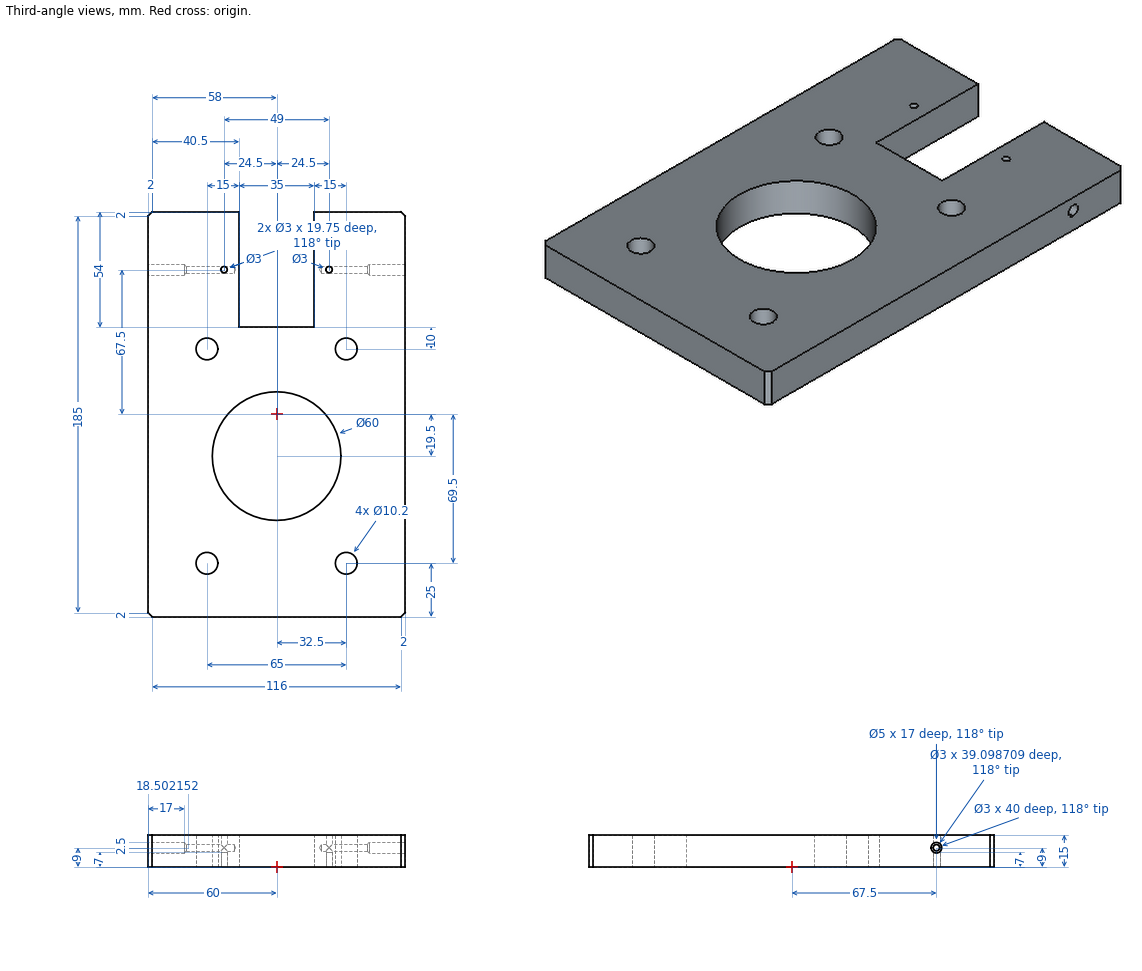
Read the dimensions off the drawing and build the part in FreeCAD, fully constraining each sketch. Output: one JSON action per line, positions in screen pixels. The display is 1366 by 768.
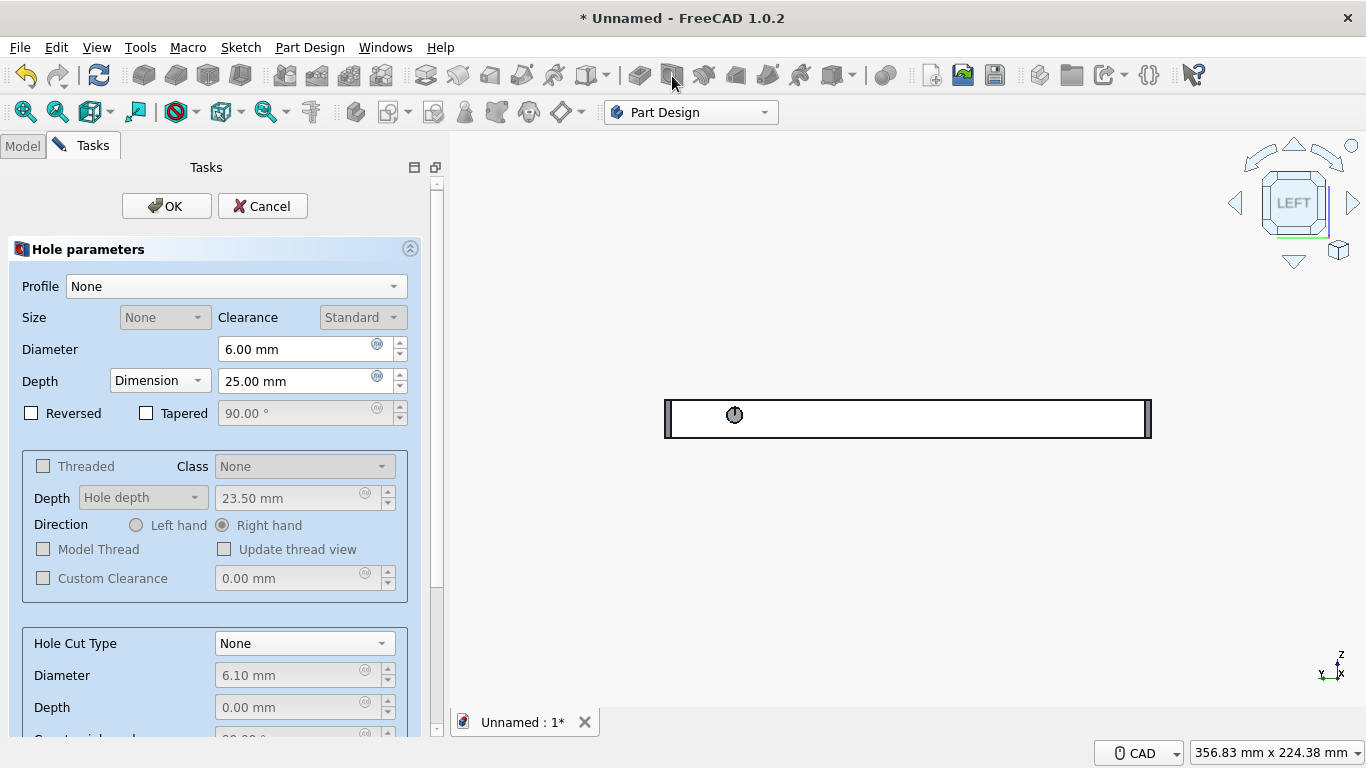
{"action": "triple_click", "coordinate": [305, 349]}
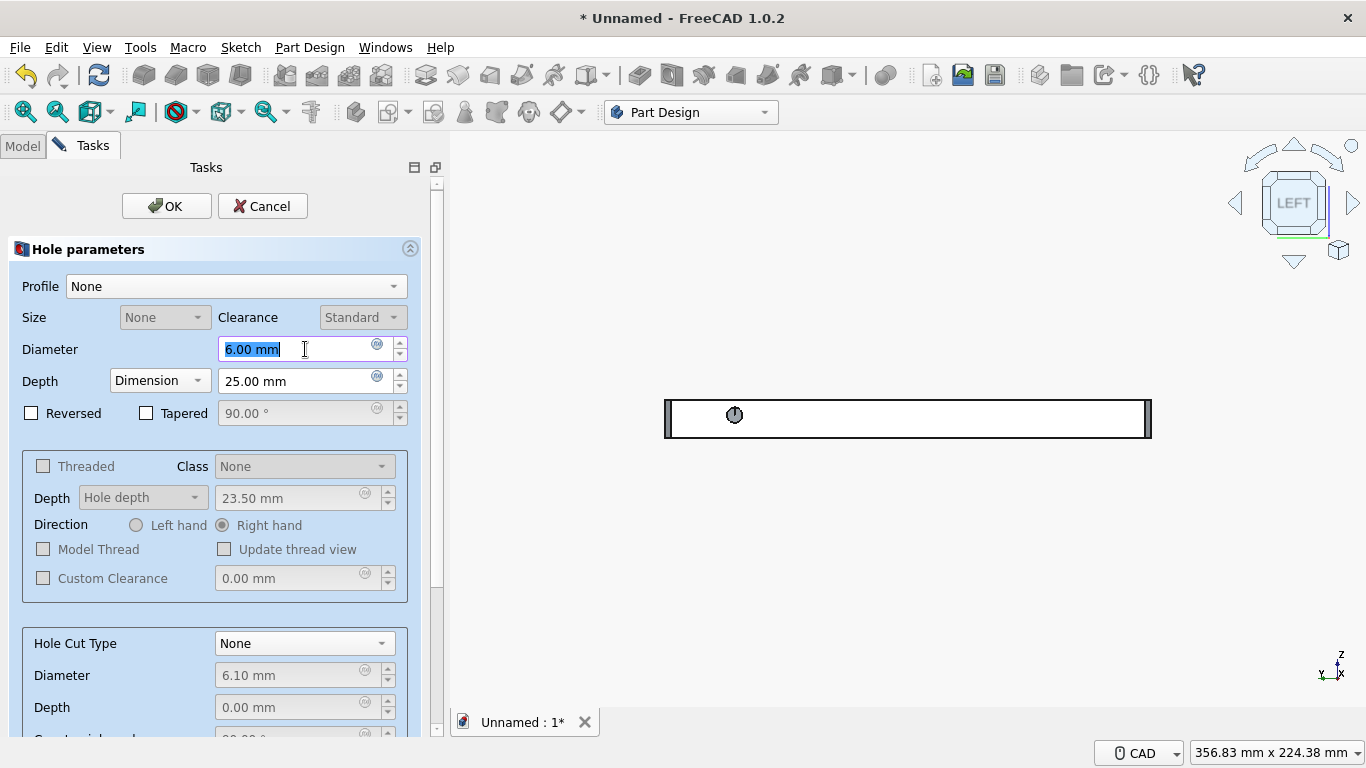
{"action": "type", "text": "3"}
{"action": "key", "text": "Tab"}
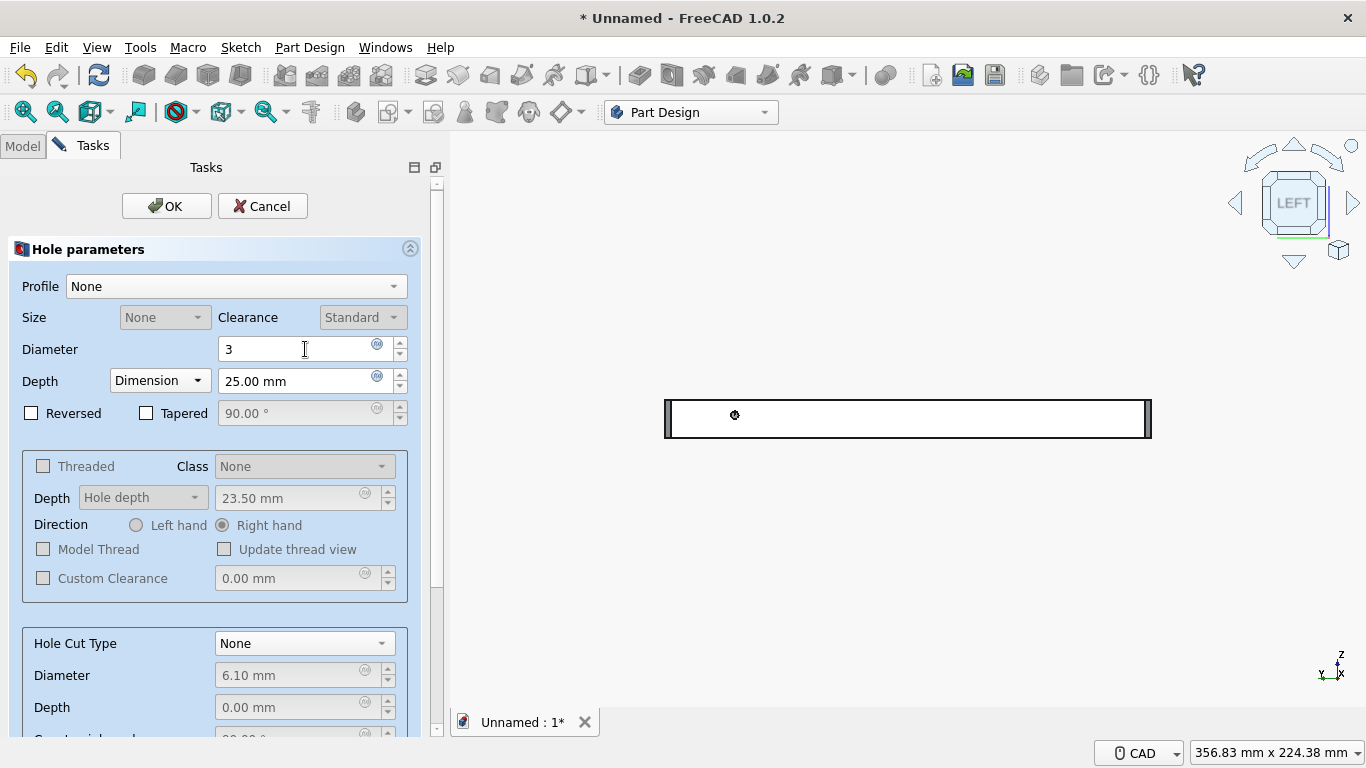
{"action": "triple_click", "coordinate": [305, 381]}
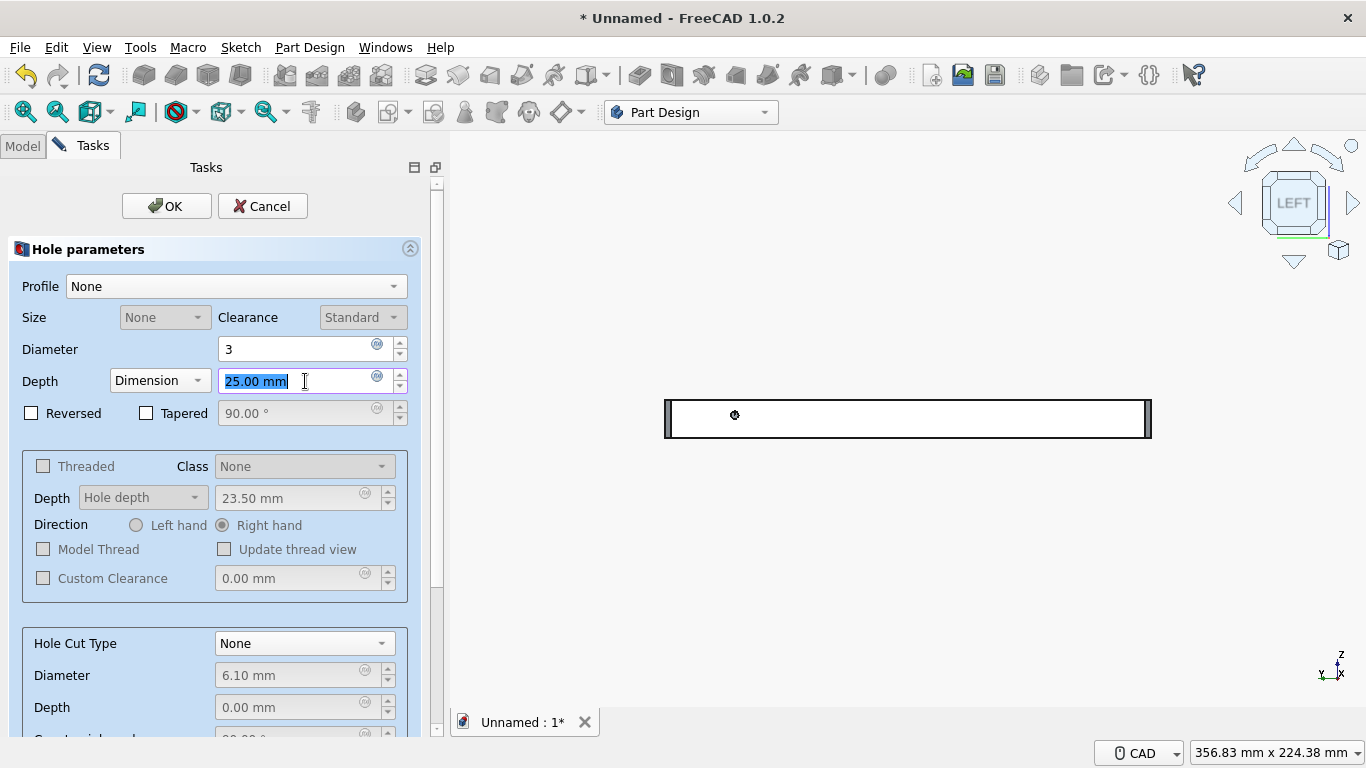
{"action": "type", "text": "40"}
{"action": "key", "text": "Tab"}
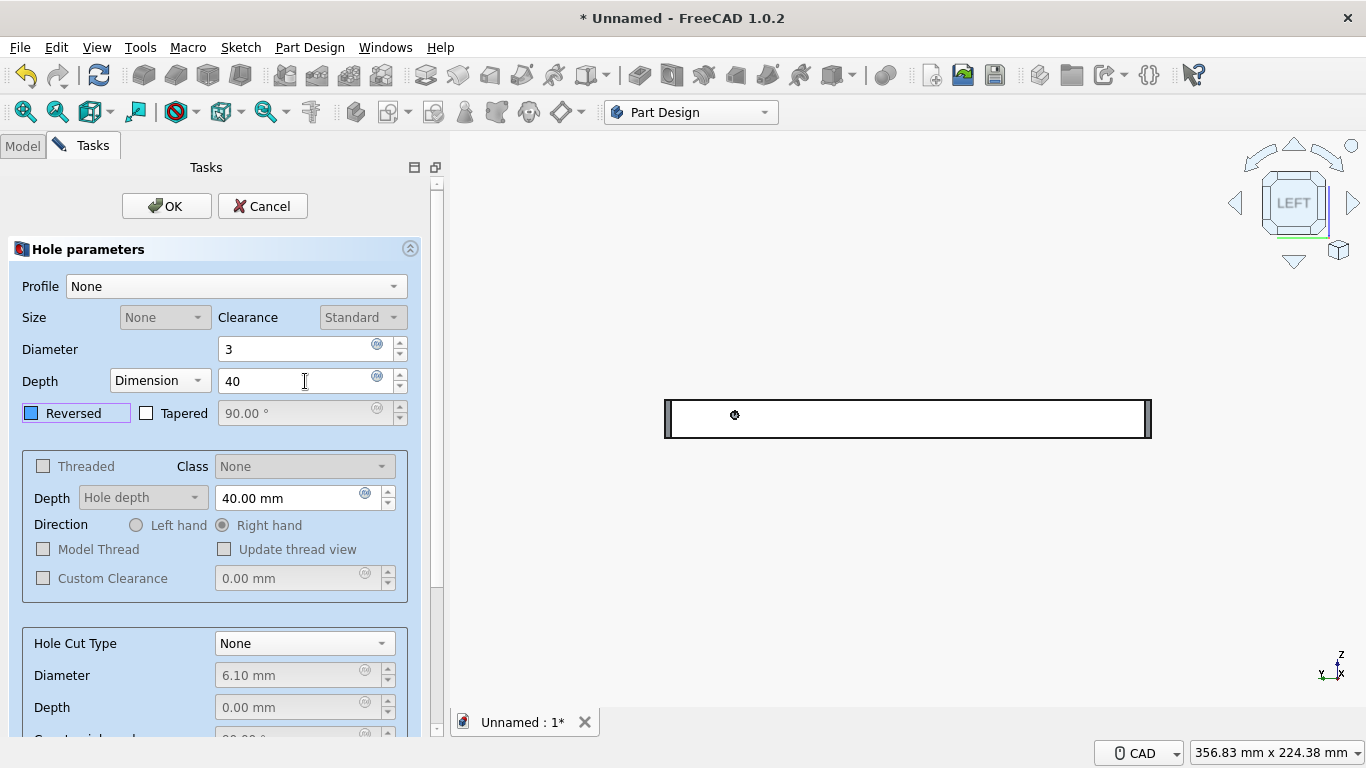
{"action": "left_click", "coordinate": [167, 206]}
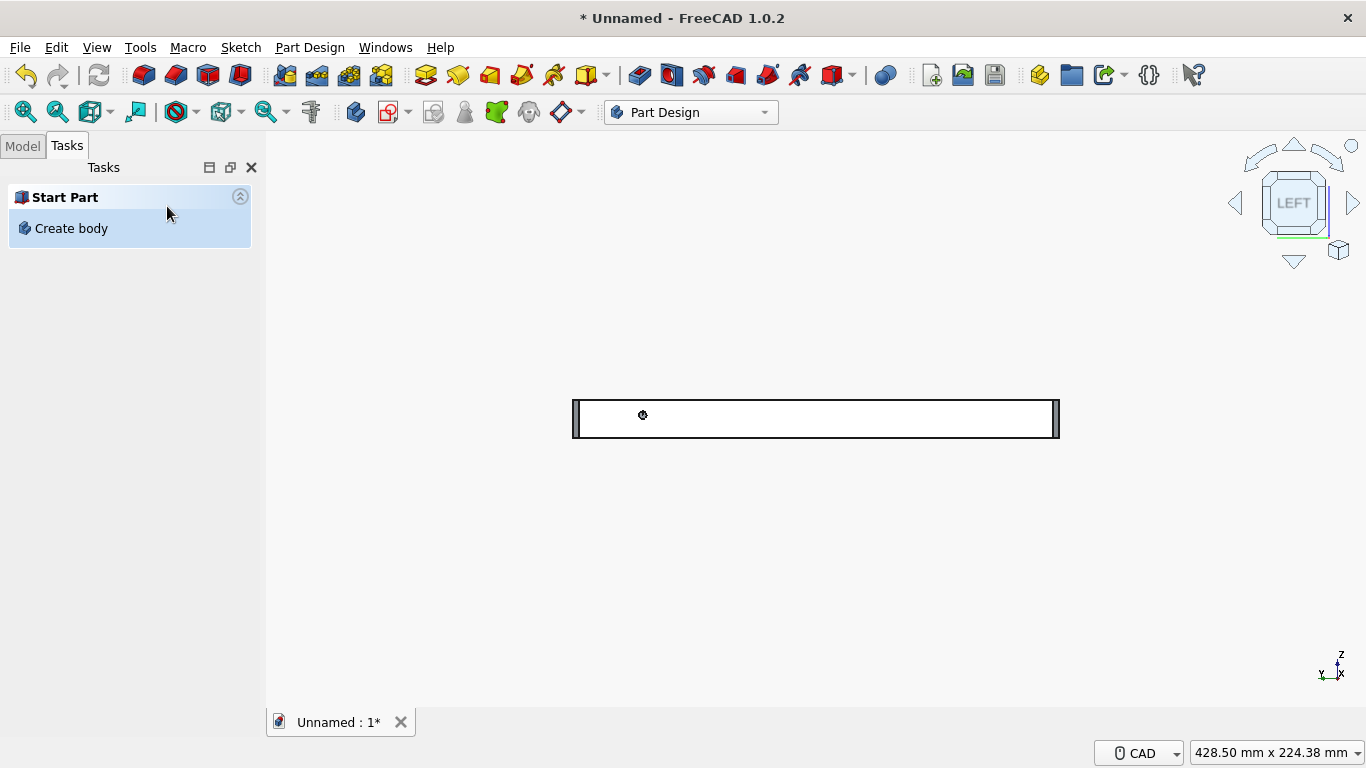
{"action": "key", "text": "v f"}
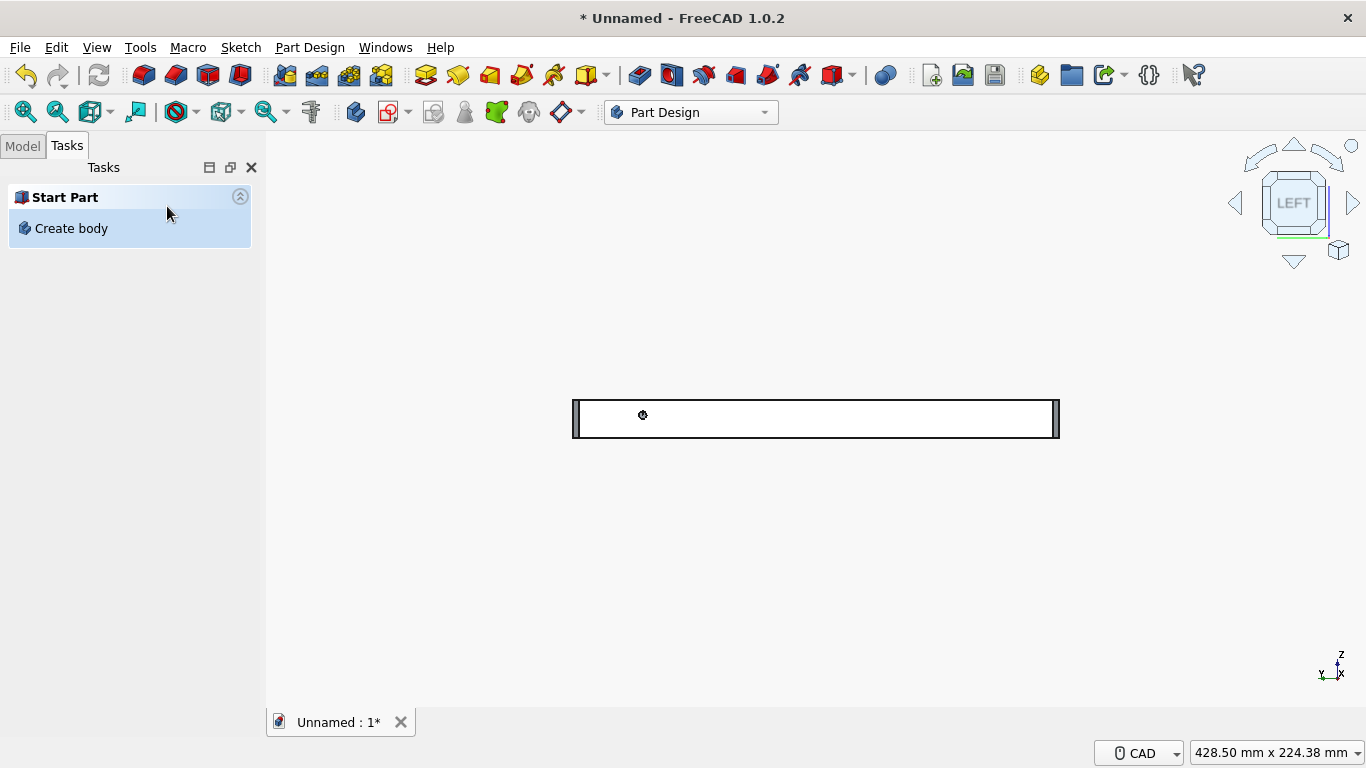
{"action": "left_click", "coordinate": [23, 145]}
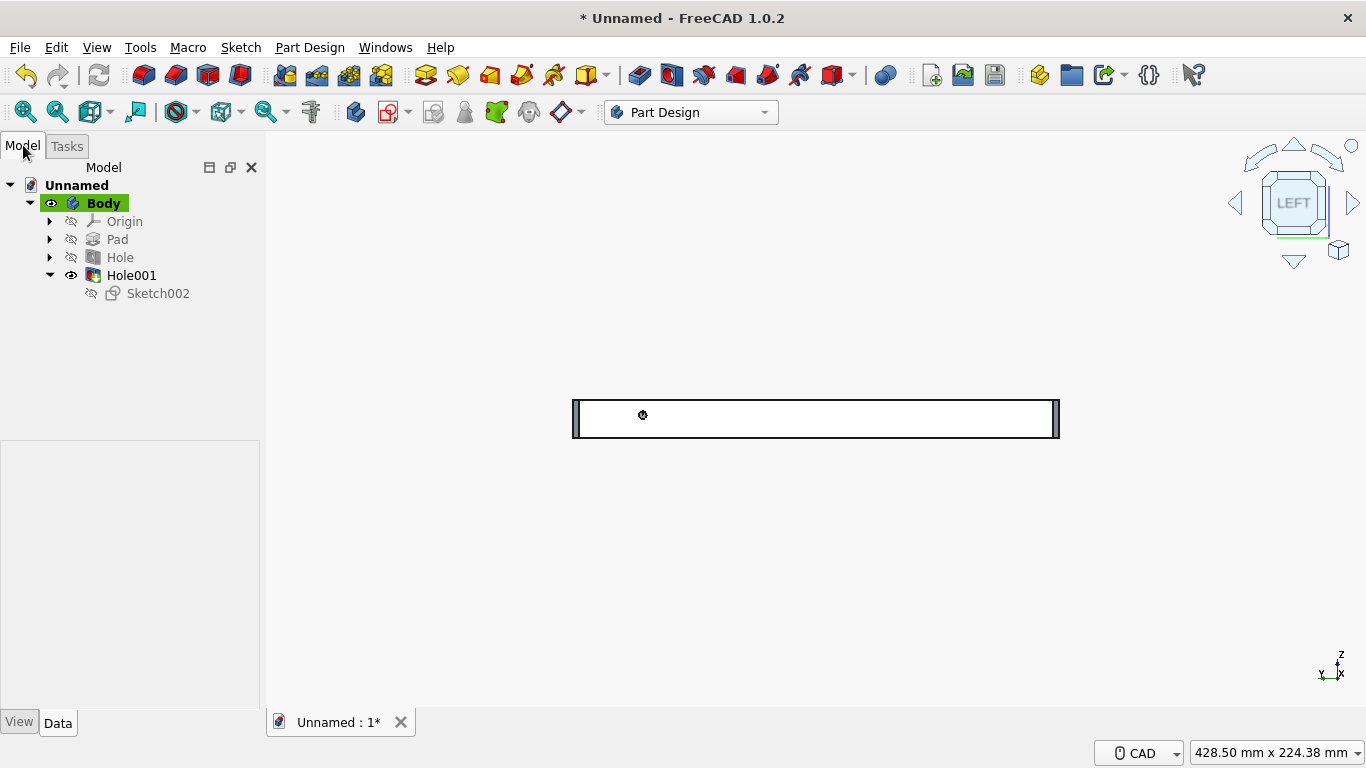
{"action": "left_click", "coordinate": [50, 221]}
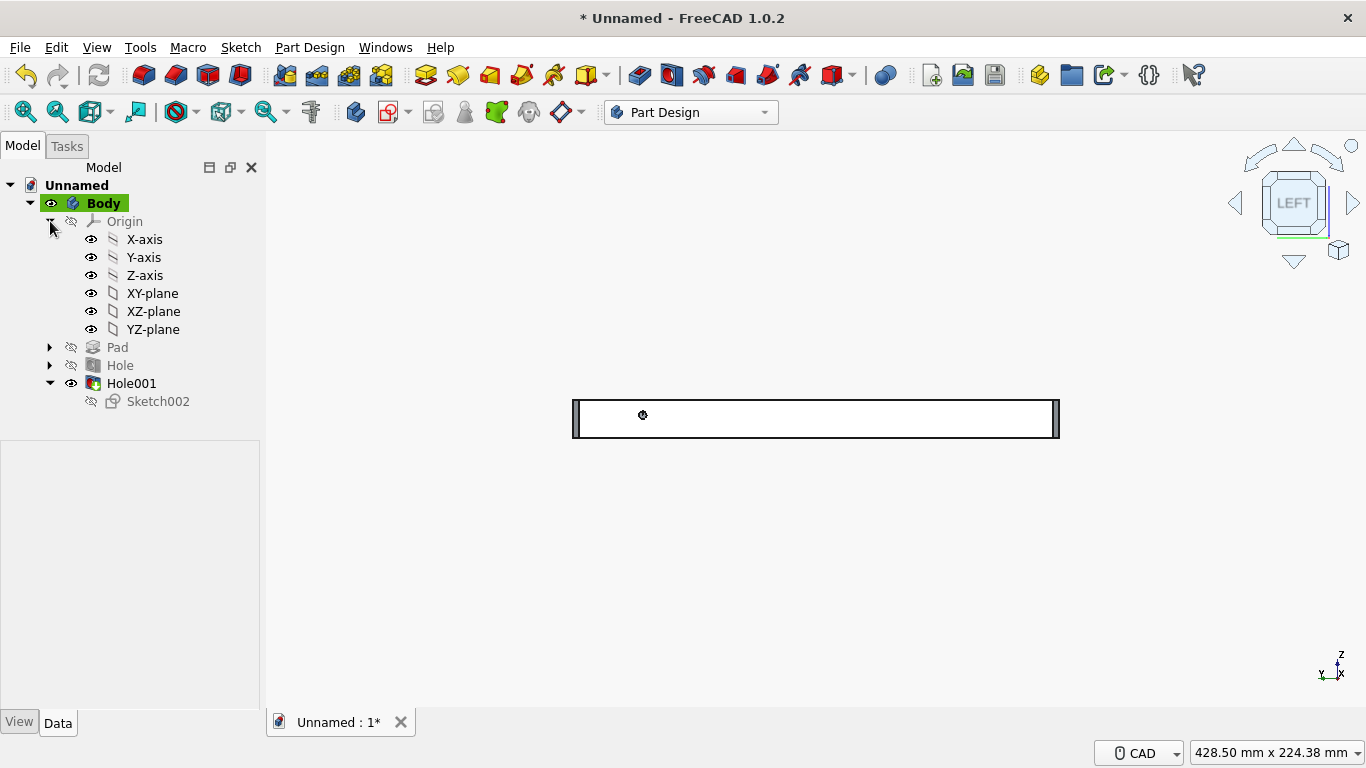
{"action": "left_click", "coordinate": [136, 311]}